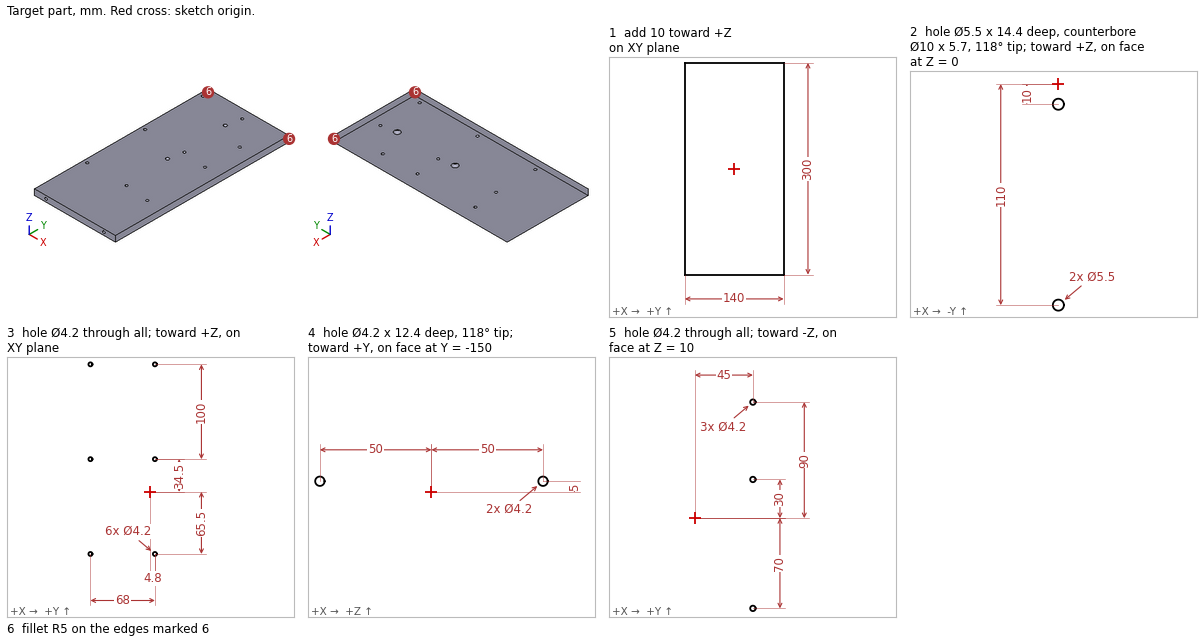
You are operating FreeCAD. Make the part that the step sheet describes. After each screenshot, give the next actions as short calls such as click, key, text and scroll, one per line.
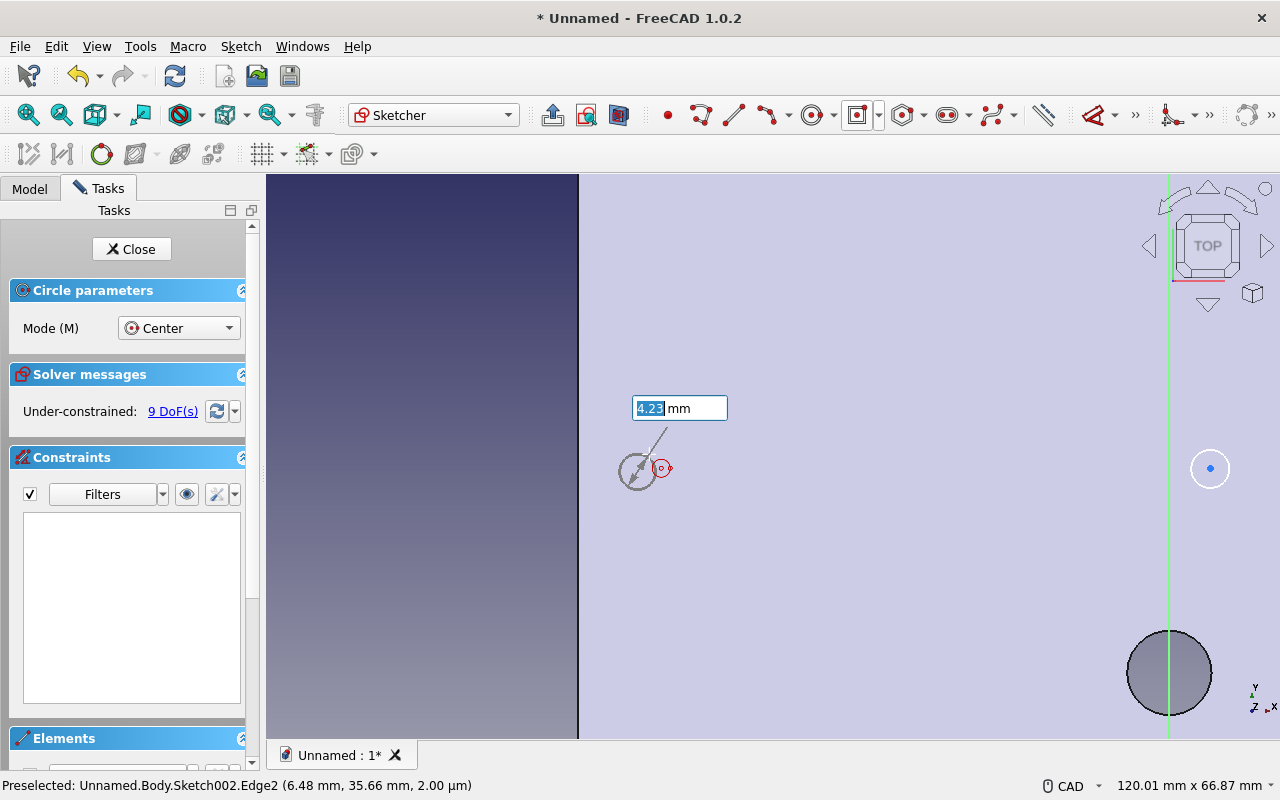
click(648, 453)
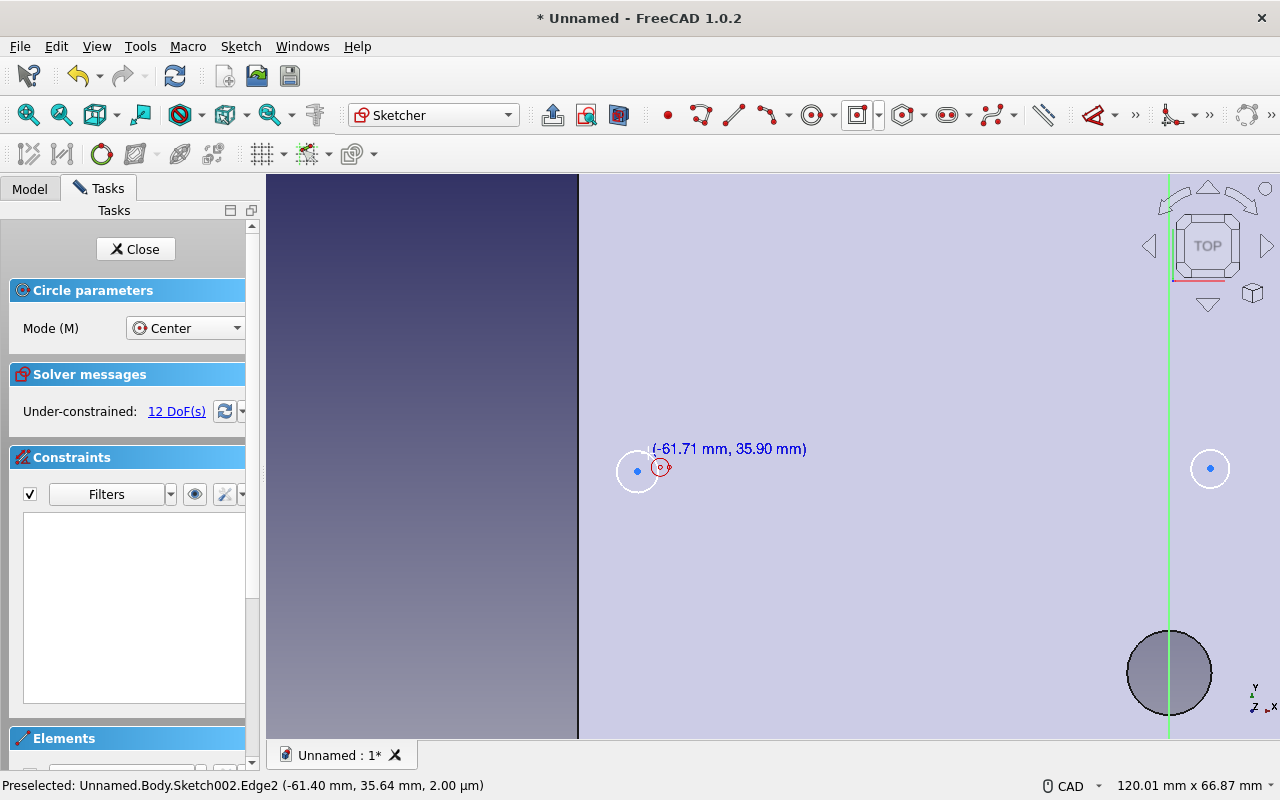
scroll(649, 454, down, 8)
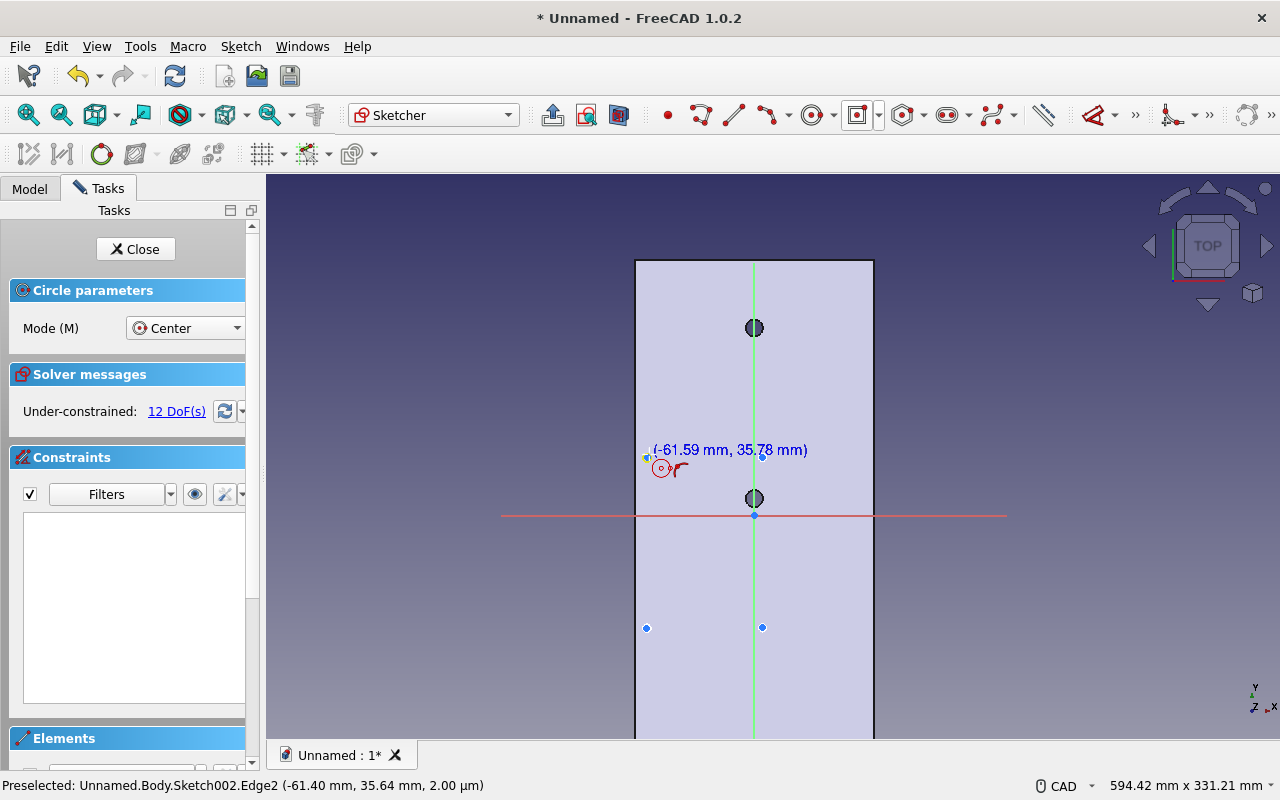
scroll(763, 286, up, 10)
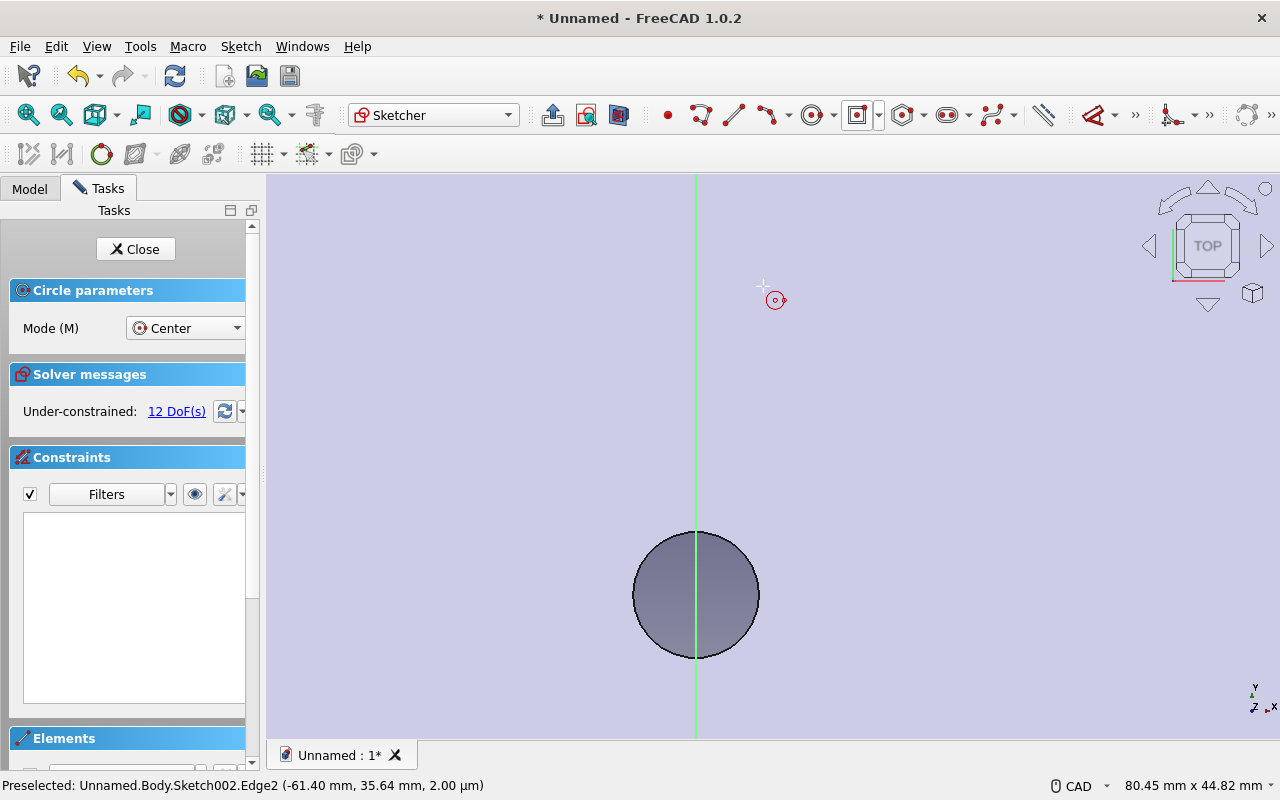
scroll(763, 286, down, 10)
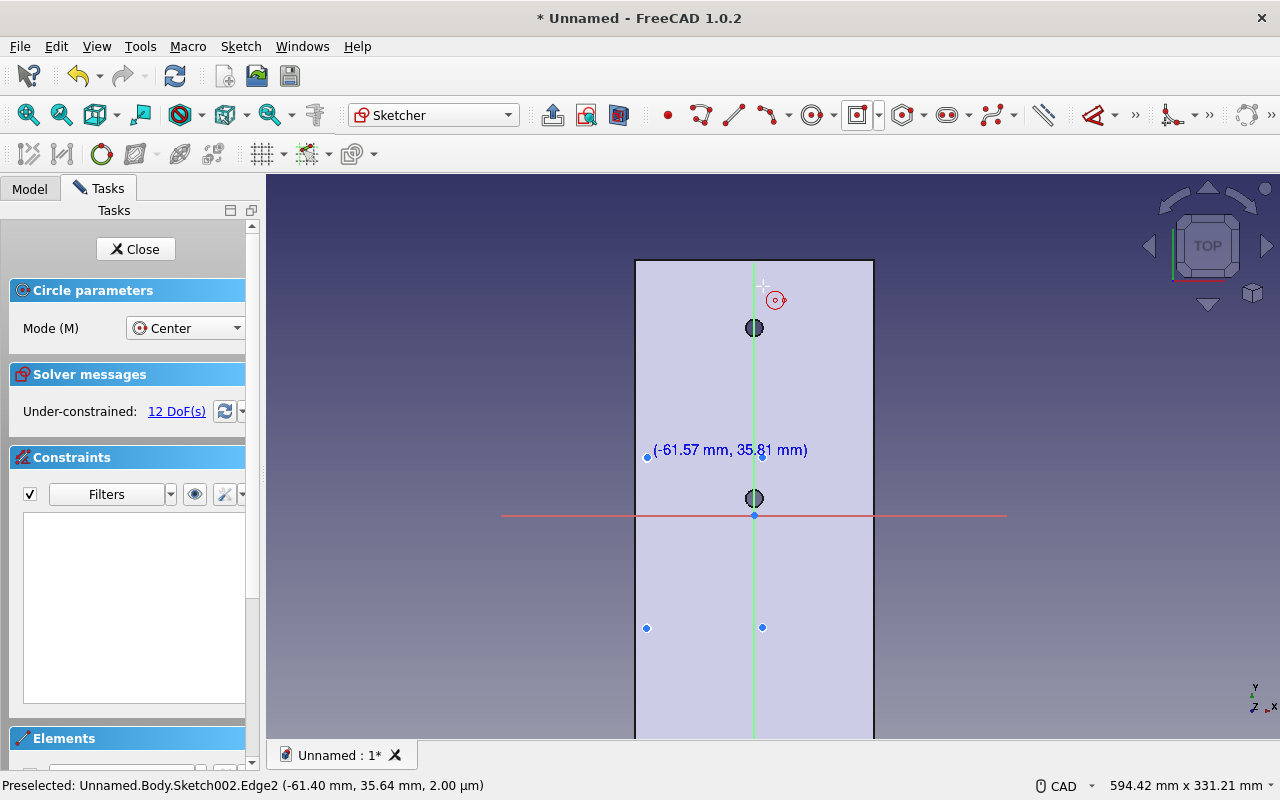
scroll(763, 286, up, 4)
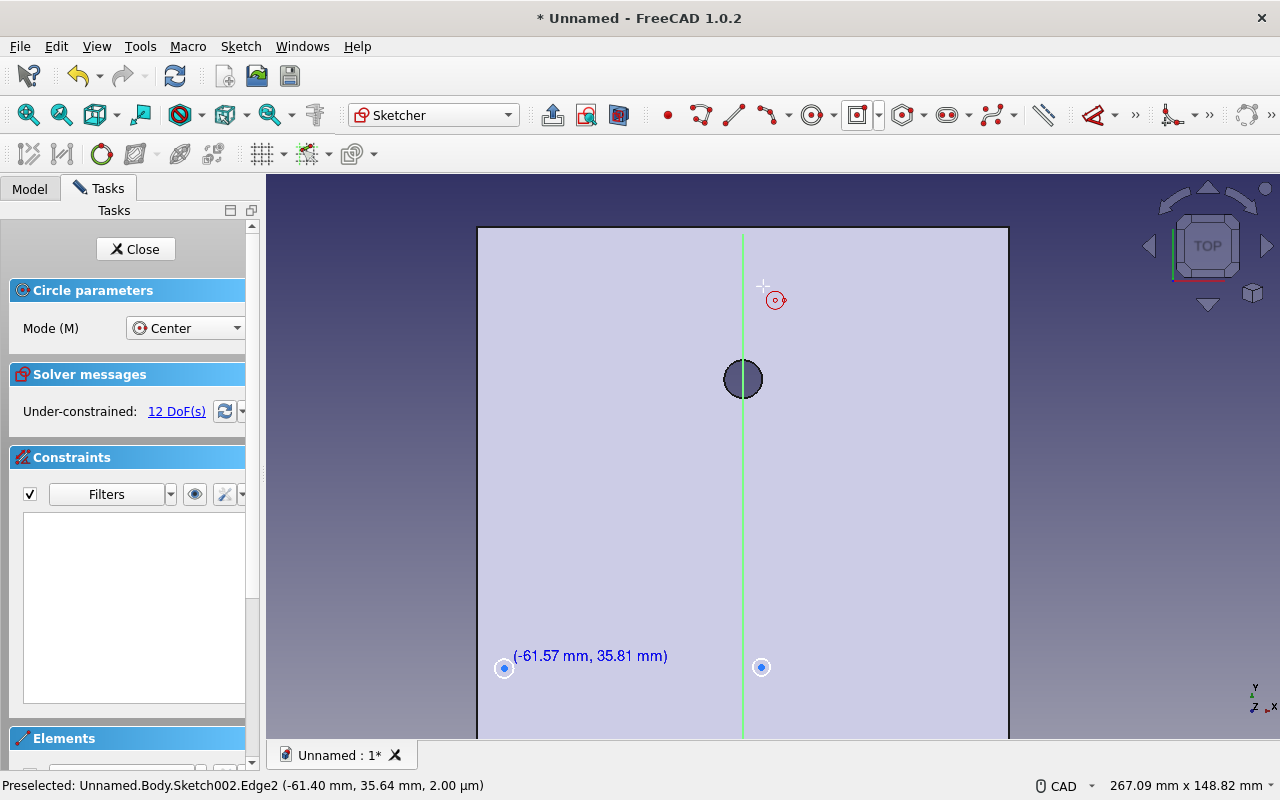
click(761, 286)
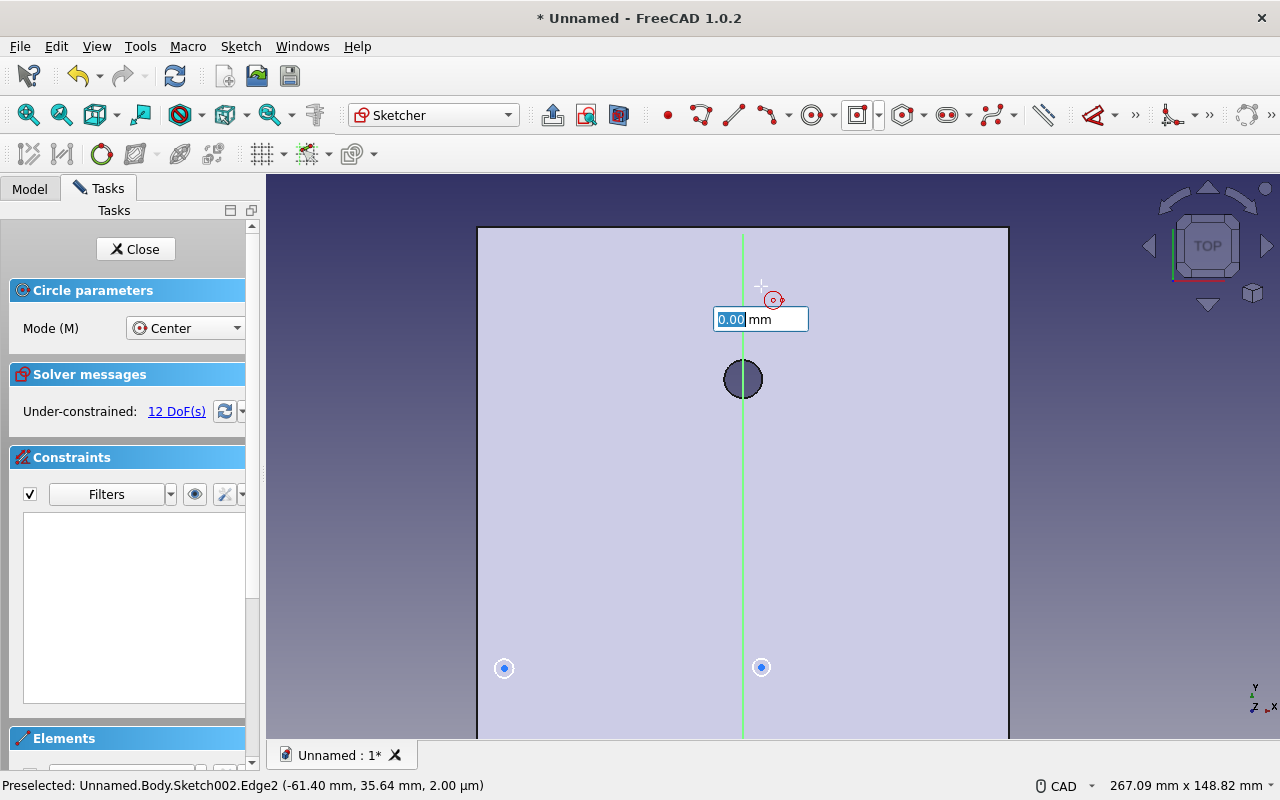
scroll(767, 281, up, 4)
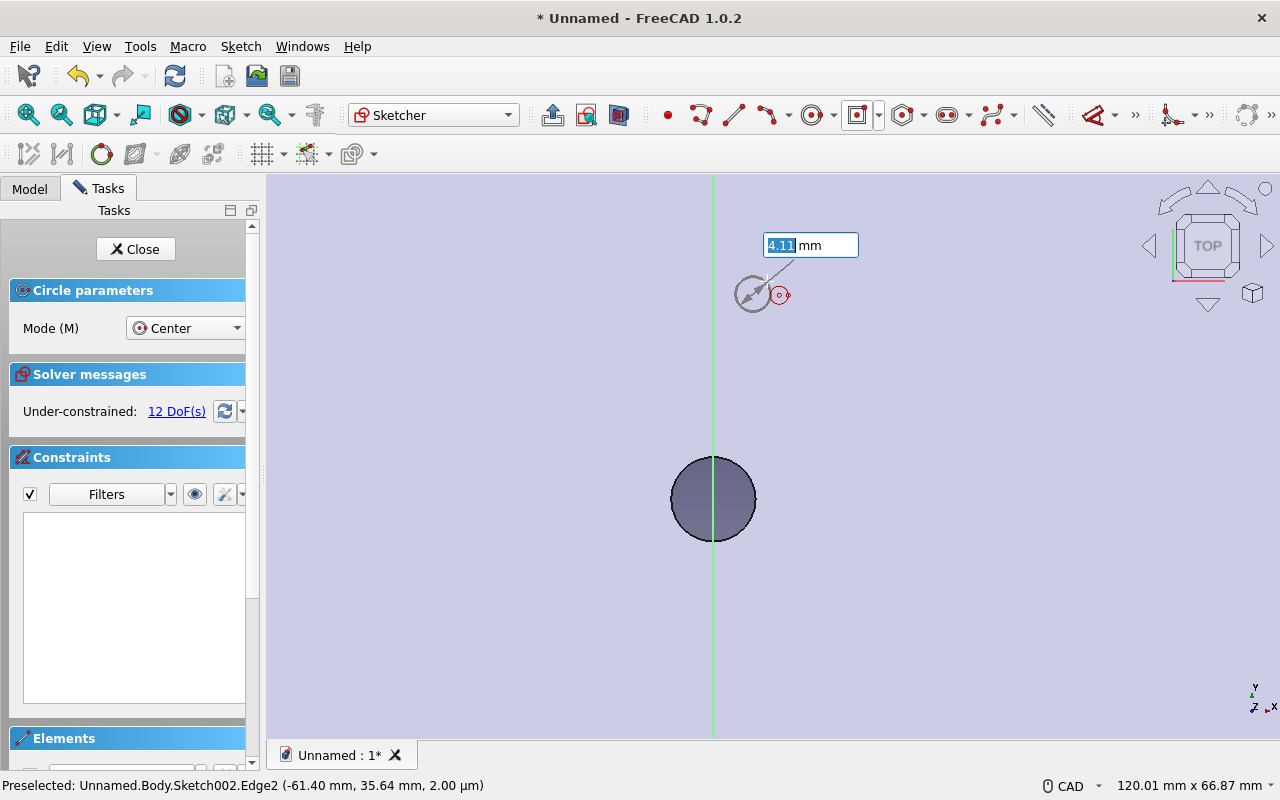
click(766, 280)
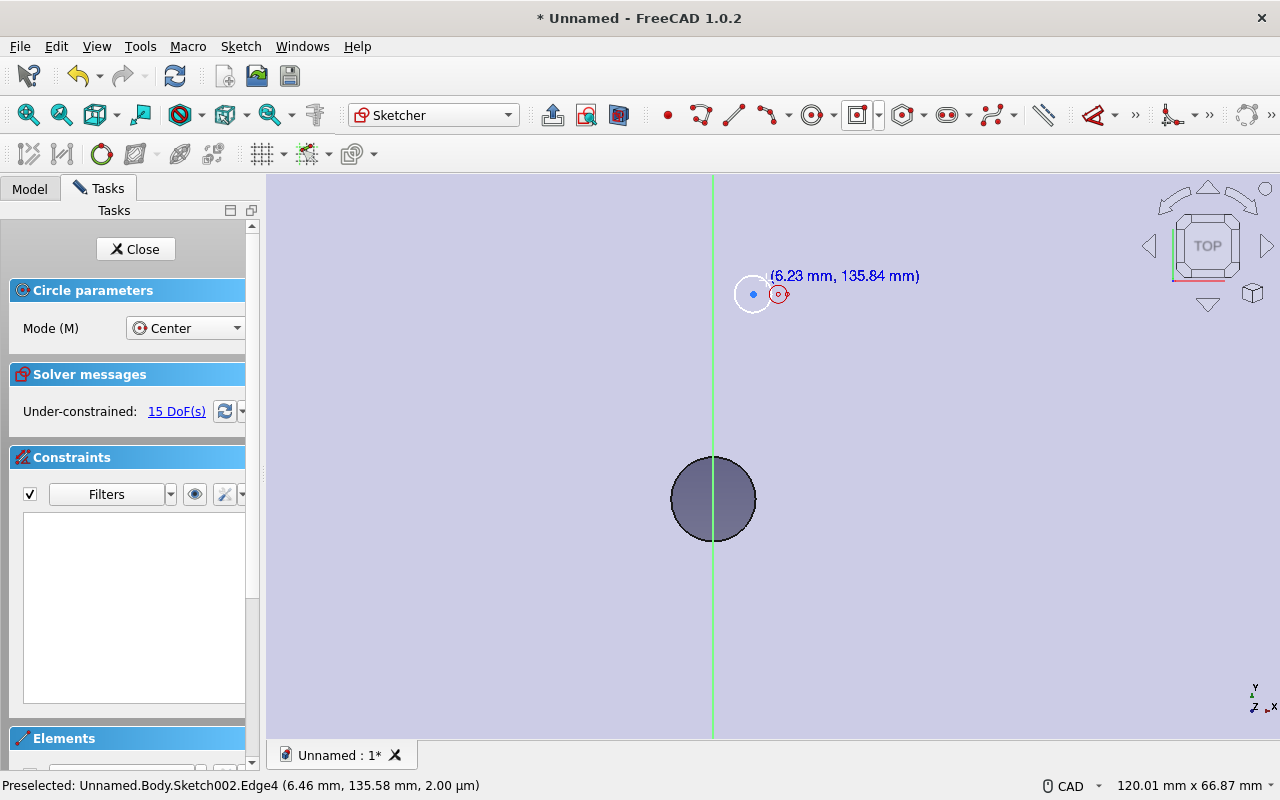
scroll(765, 284, down, 8)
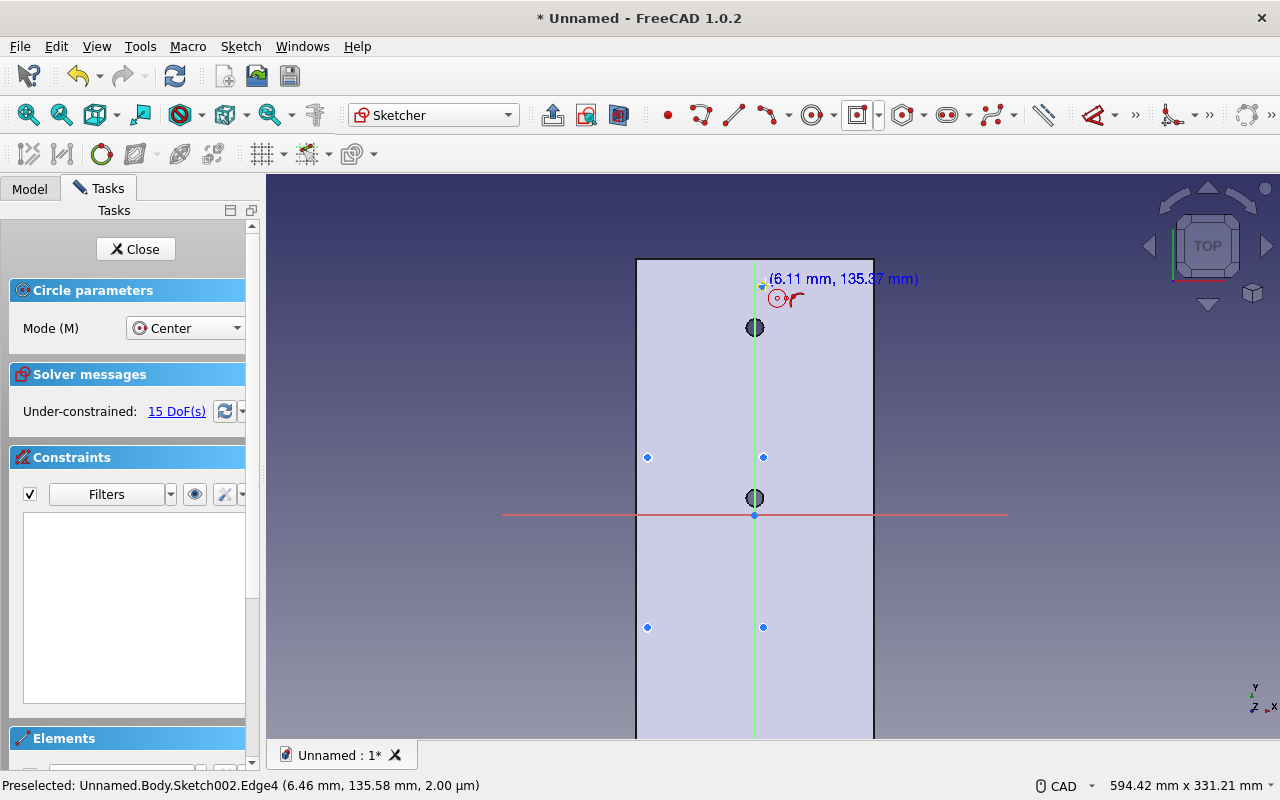
scroll(647, 286, up, 10)